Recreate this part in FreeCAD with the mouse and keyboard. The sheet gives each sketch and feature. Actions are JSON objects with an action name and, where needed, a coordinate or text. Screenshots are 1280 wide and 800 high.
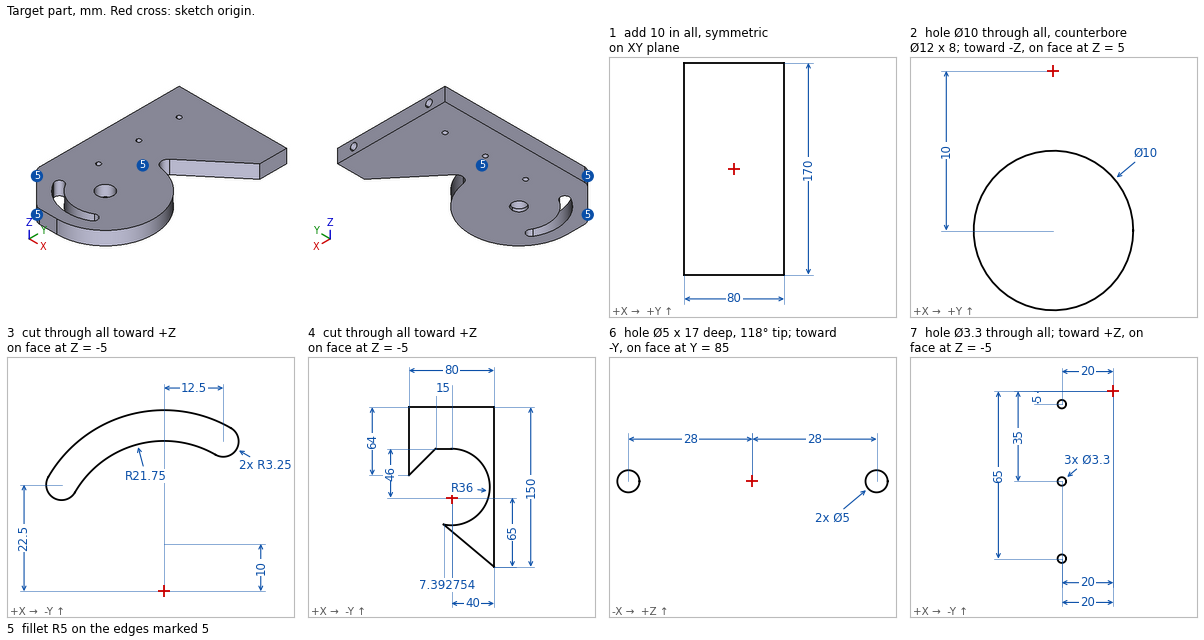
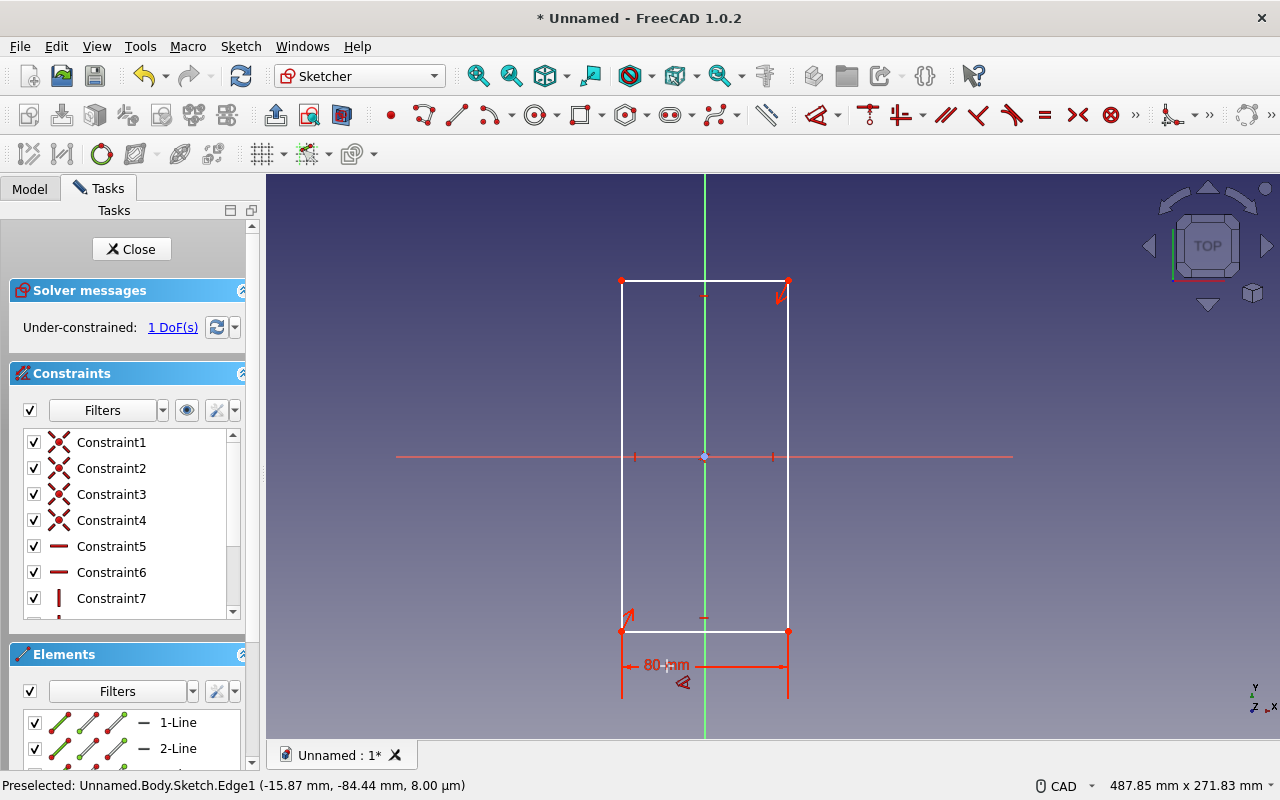
{"action": "left_click", "coordinate": [788, 527]}
{"action": "left_click", "coordinate": [822, 376]}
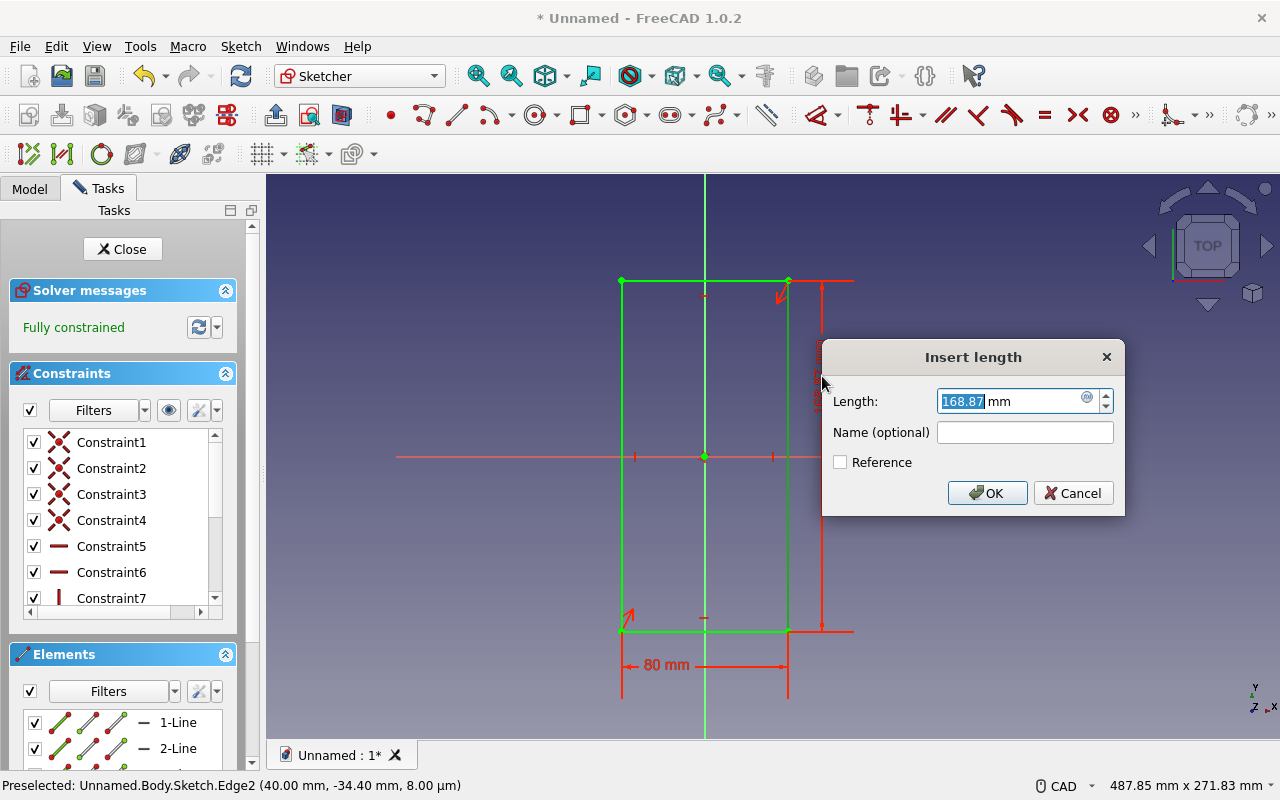
{"action": "type", "text": "170"}
{"action": "key", "text": "Return"}
{"action": "key", "text": "Escape"}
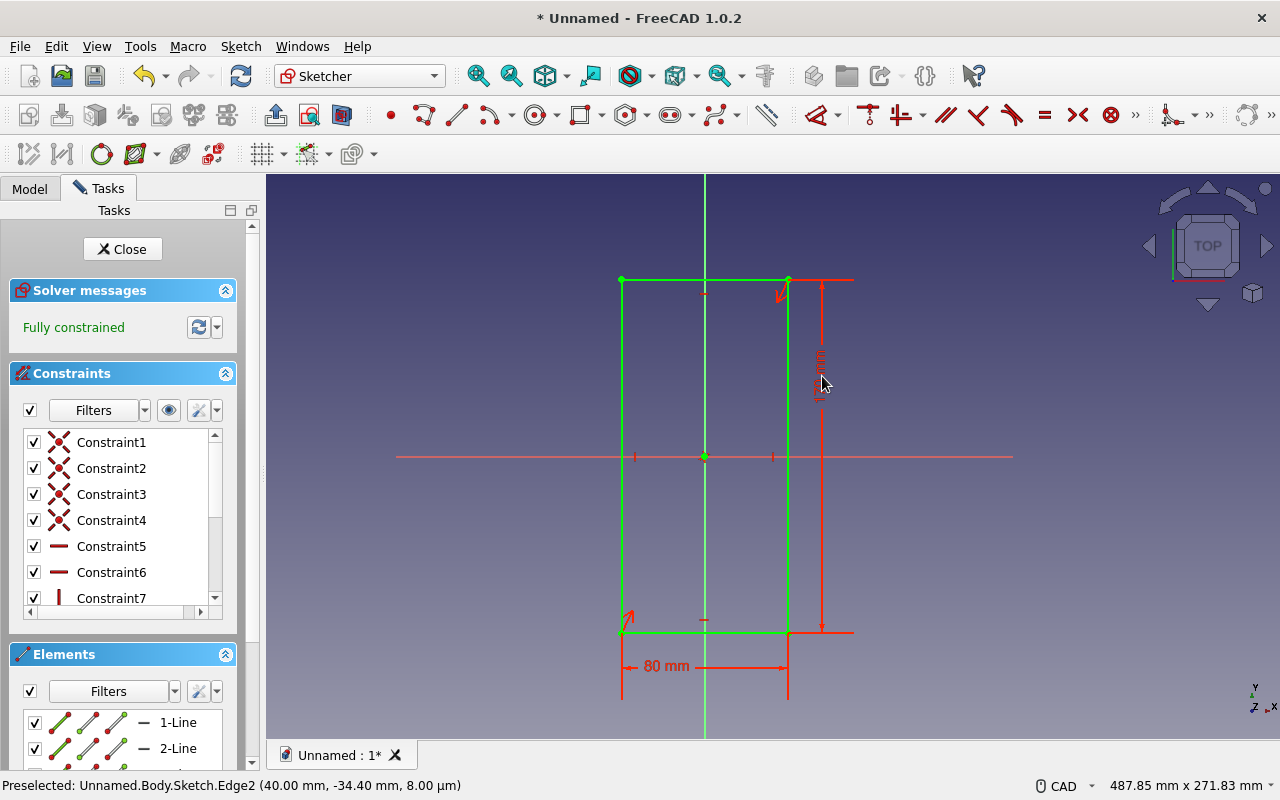
{"action": "left_click", "coordinate": [123, 249]}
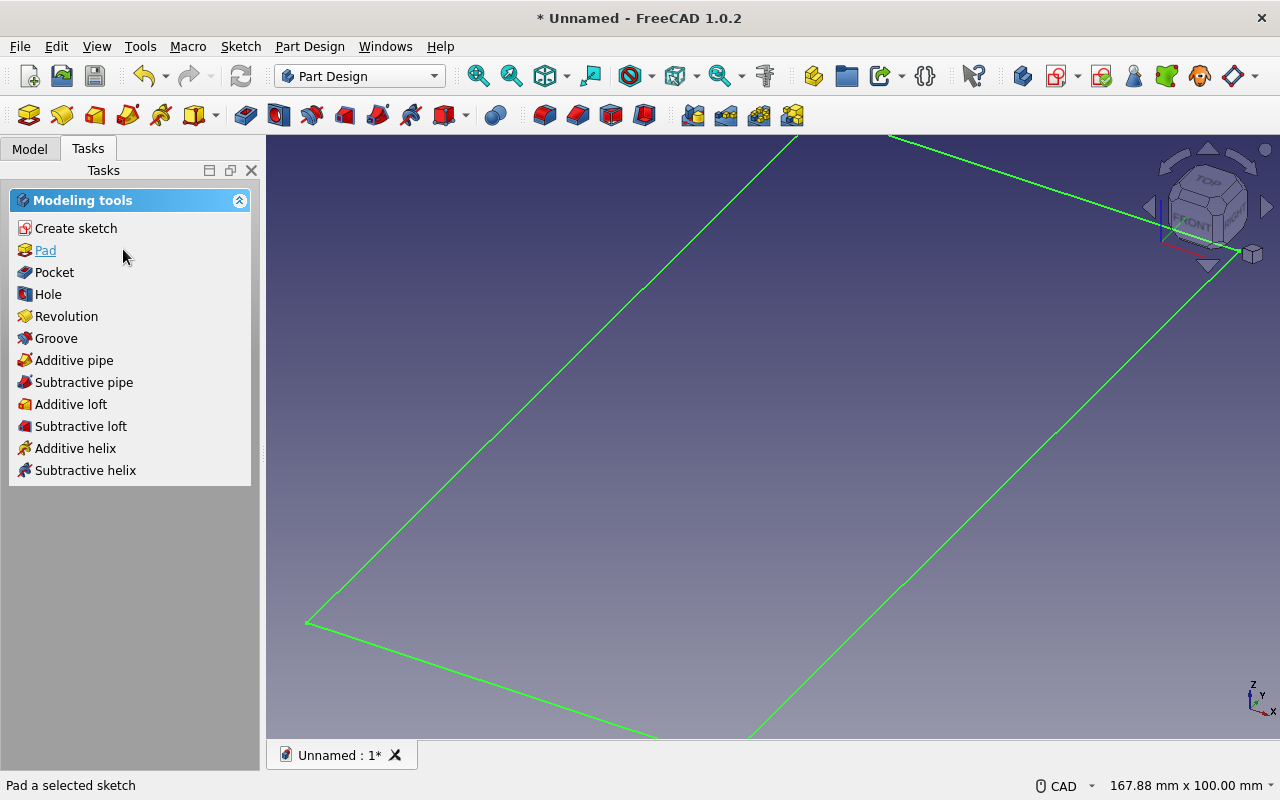
{"action": "left_click", "coordinate": [29, 116]}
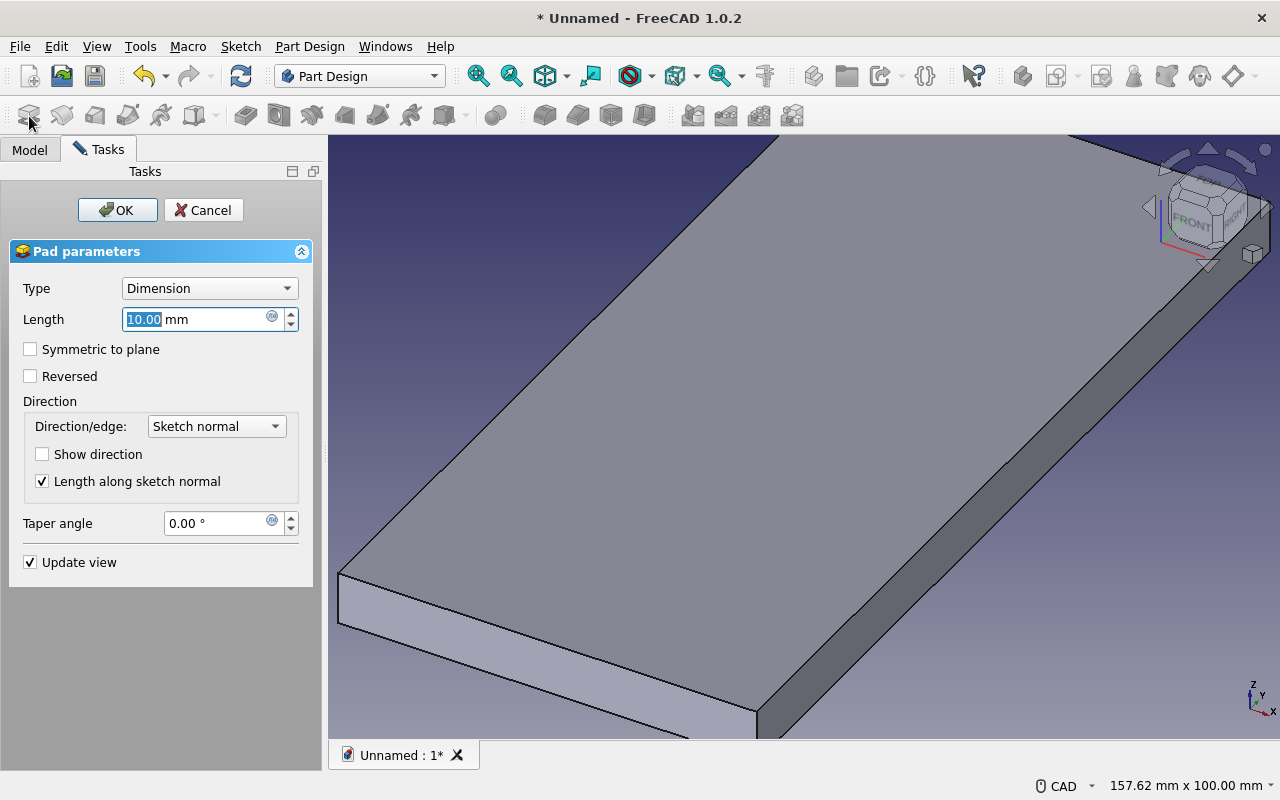
{"action": "type", "text": "10"}
{"action": "key", "text": "Tab"}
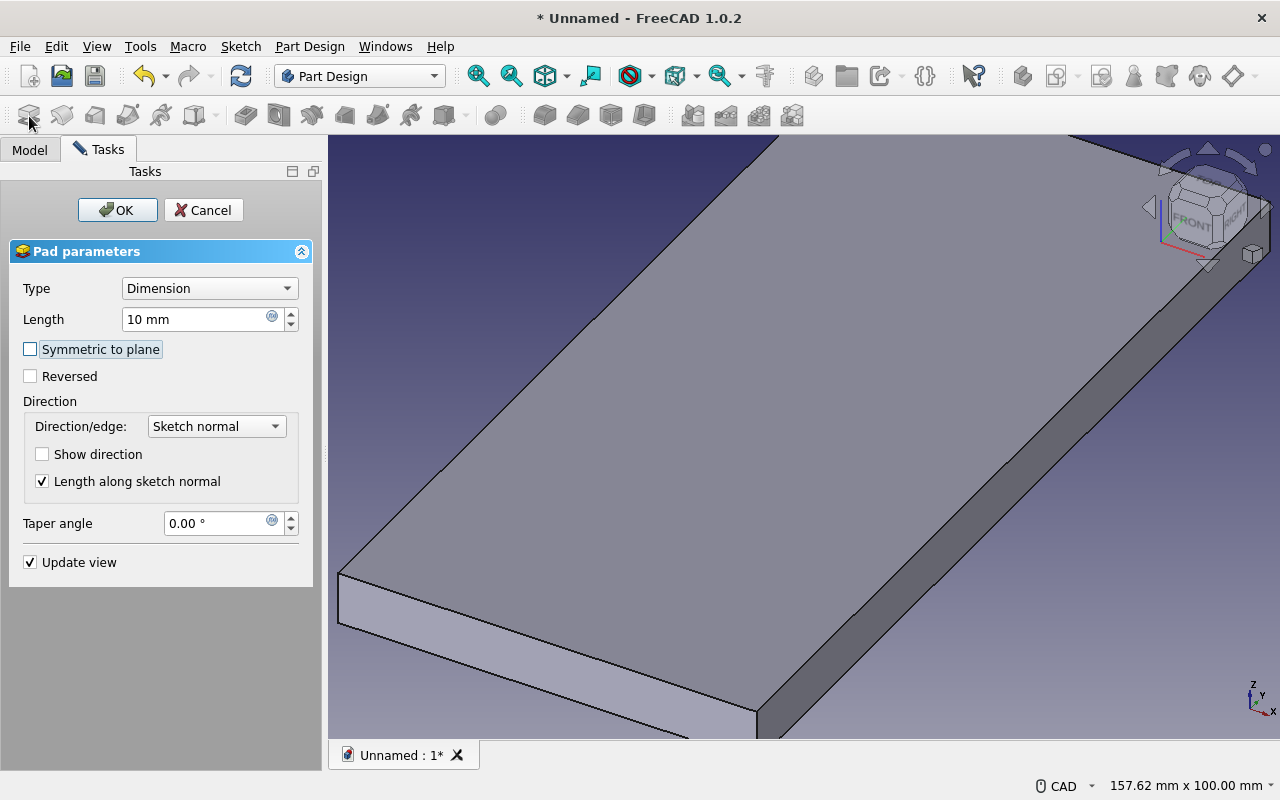
{"action": "left_click", "coordinate": [31, 349]}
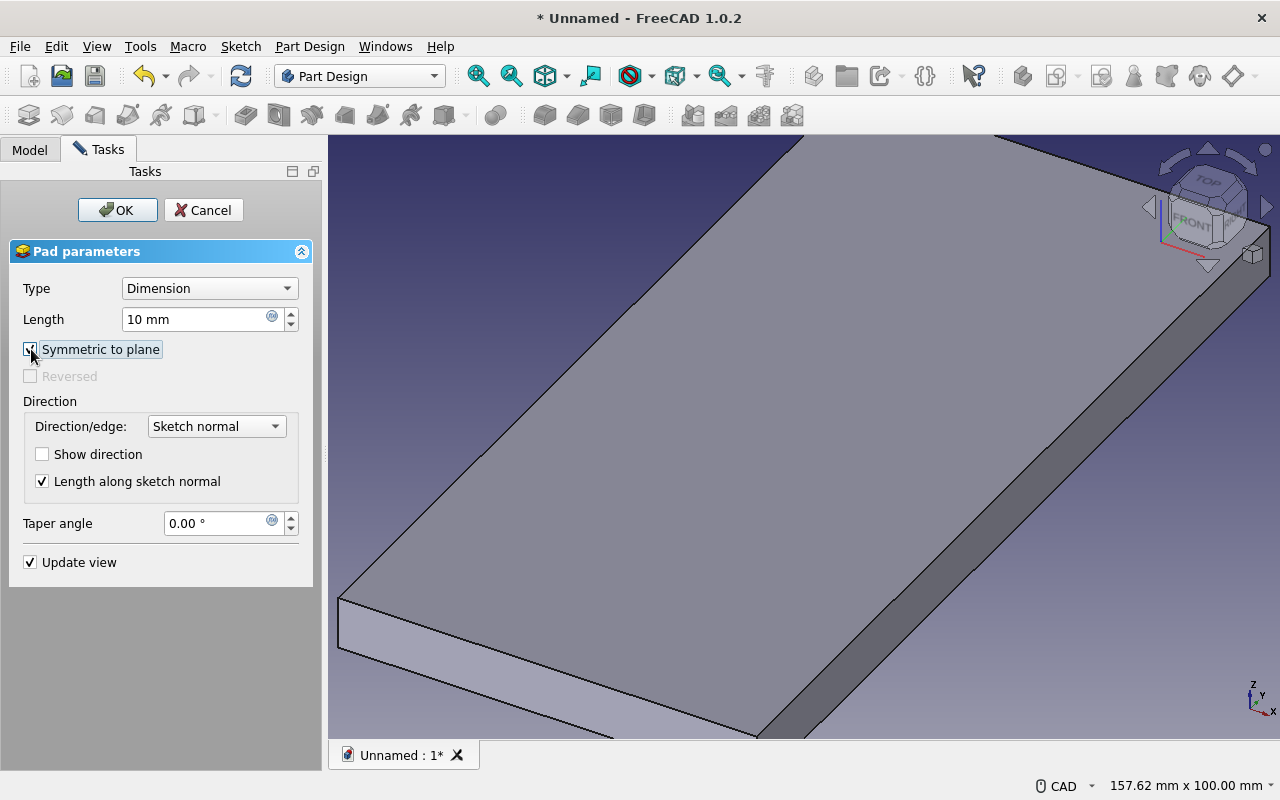
{"action": "left_click", "coordinate": [118, 210]}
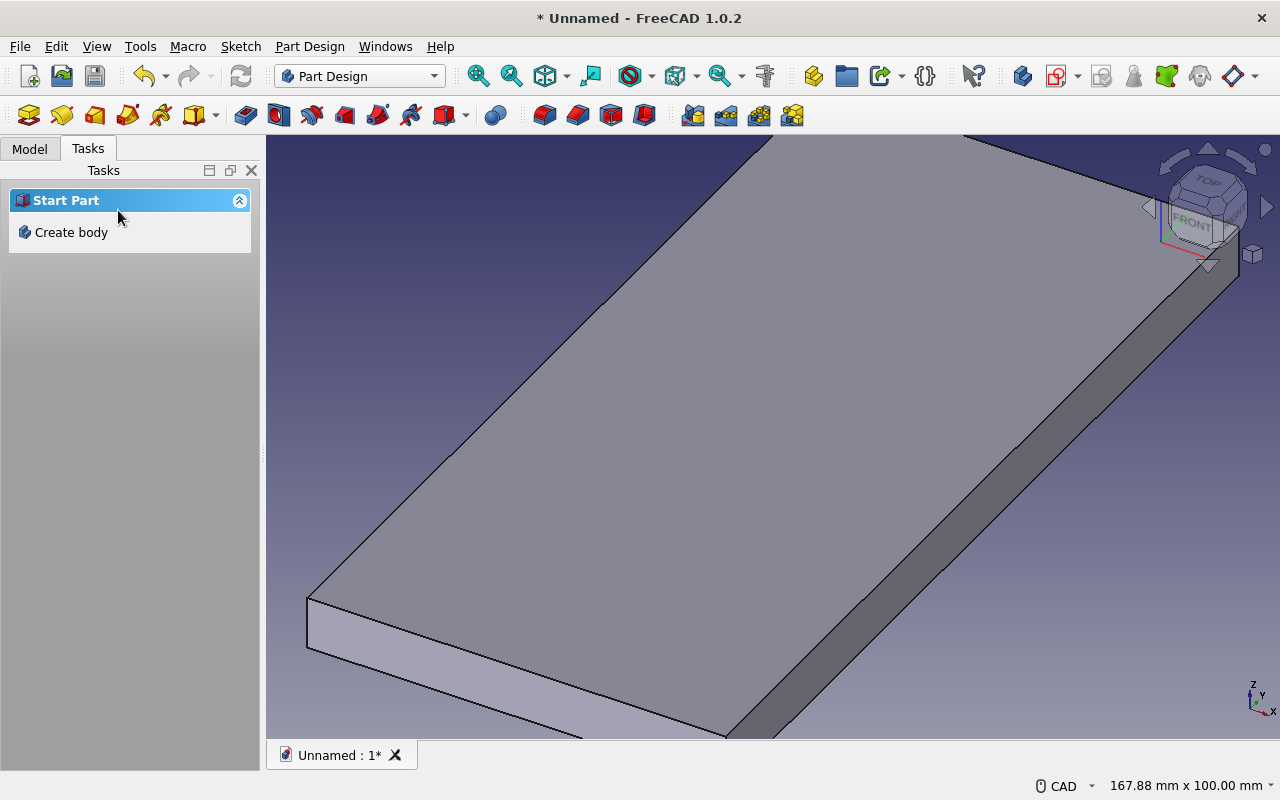
{"action": "key", "text": "v f"}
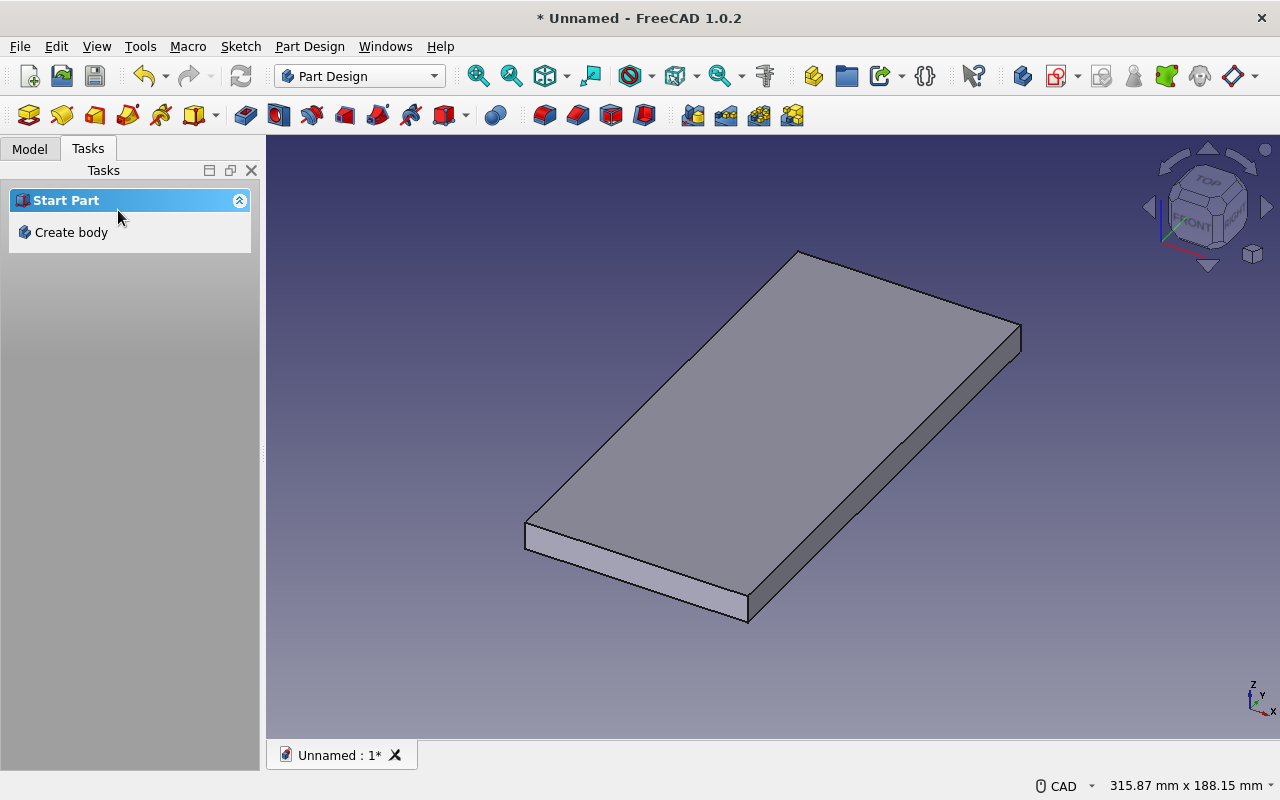
{"action": "left_click", "coordinate": [812, 384]}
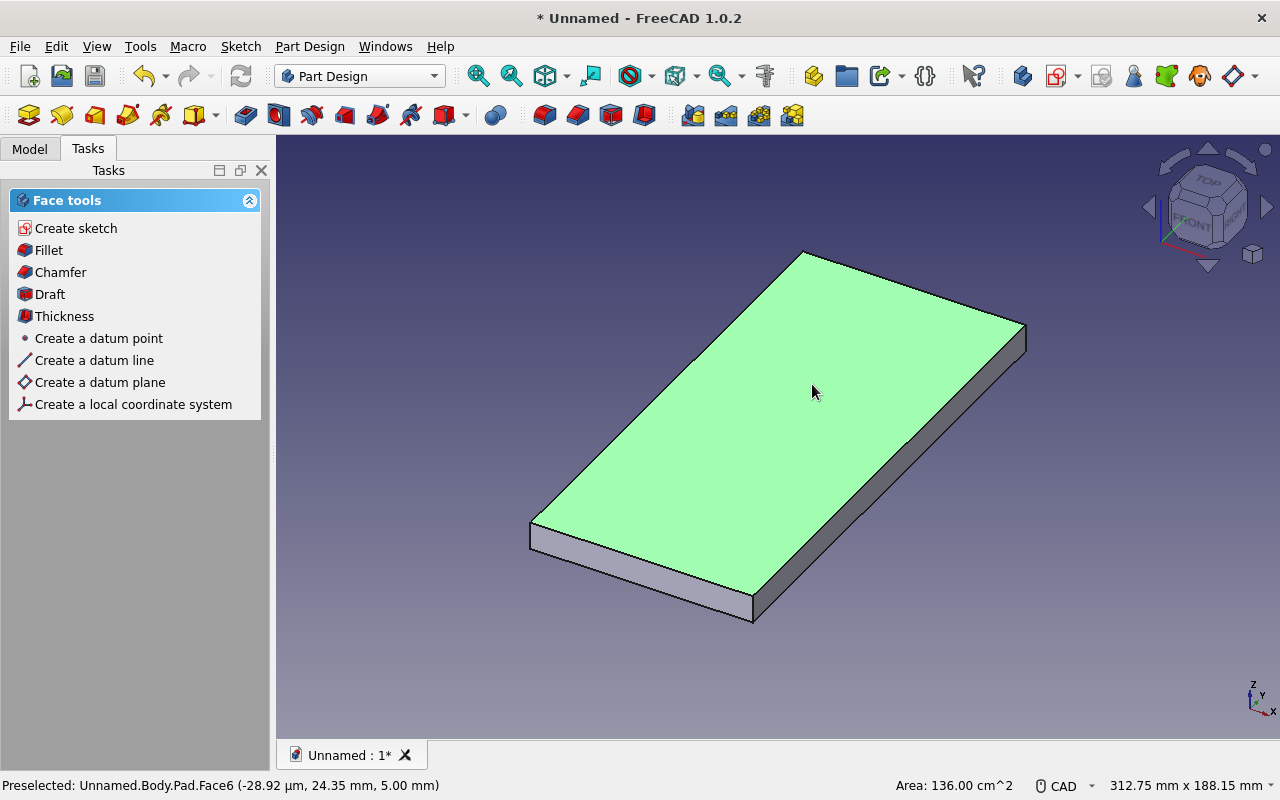
{"action": "left_click", "coordinate": [1056, 76]}